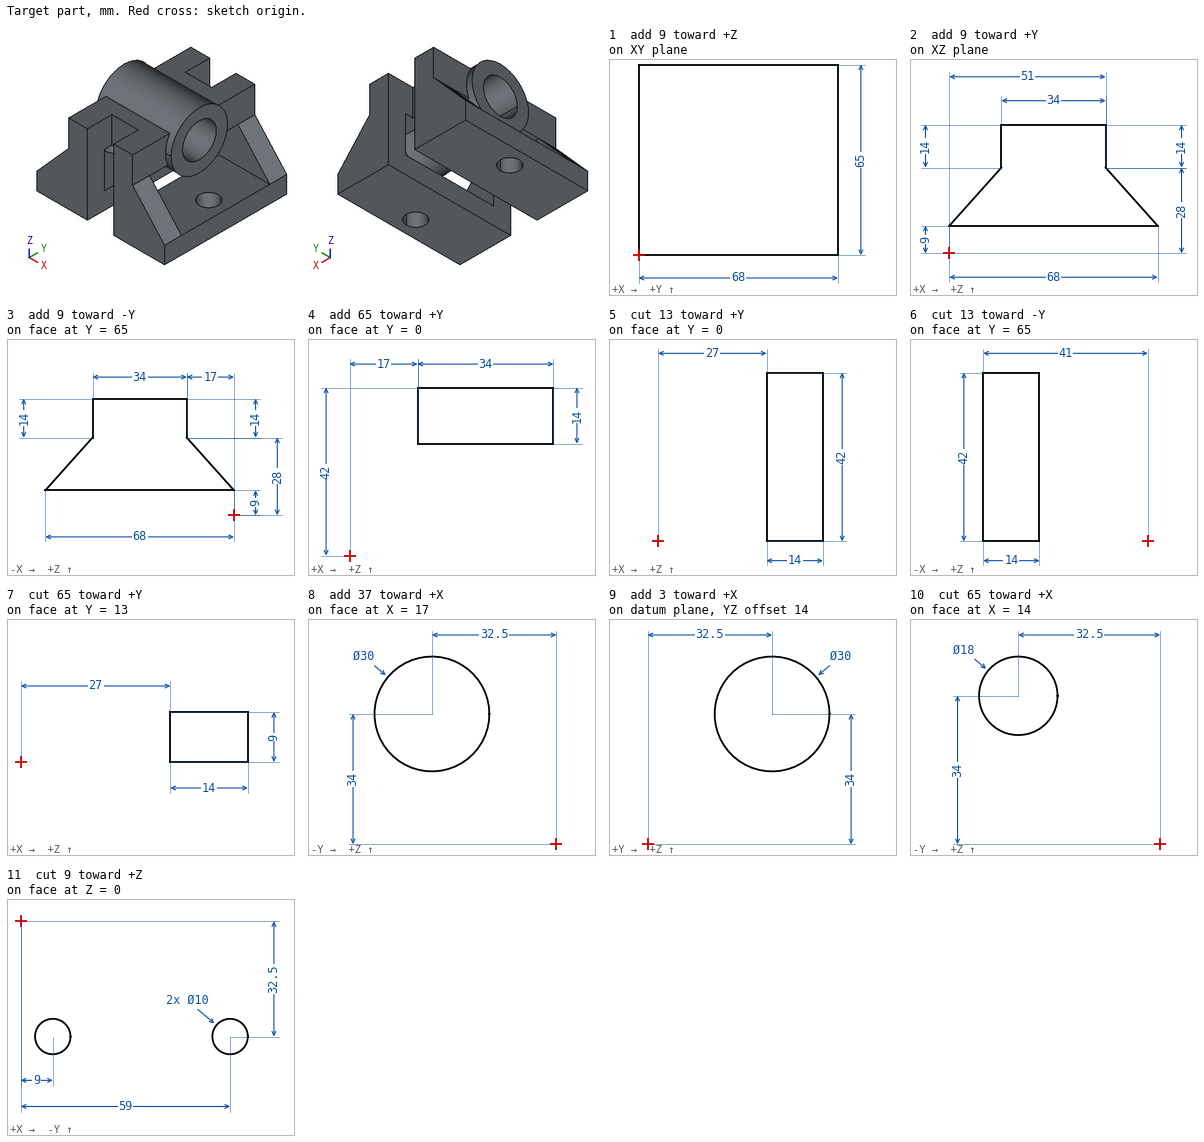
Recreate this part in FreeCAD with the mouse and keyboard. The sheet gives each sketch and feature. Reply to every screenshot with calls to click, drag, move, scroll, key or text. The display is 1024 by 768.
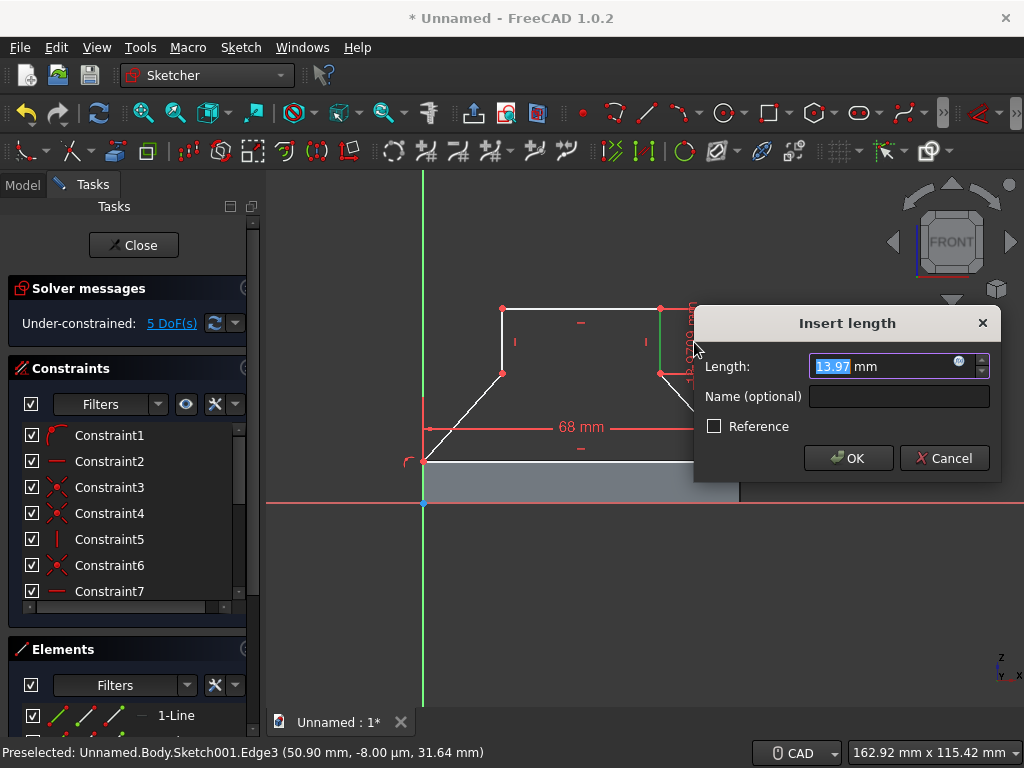
text(14)
key(Return)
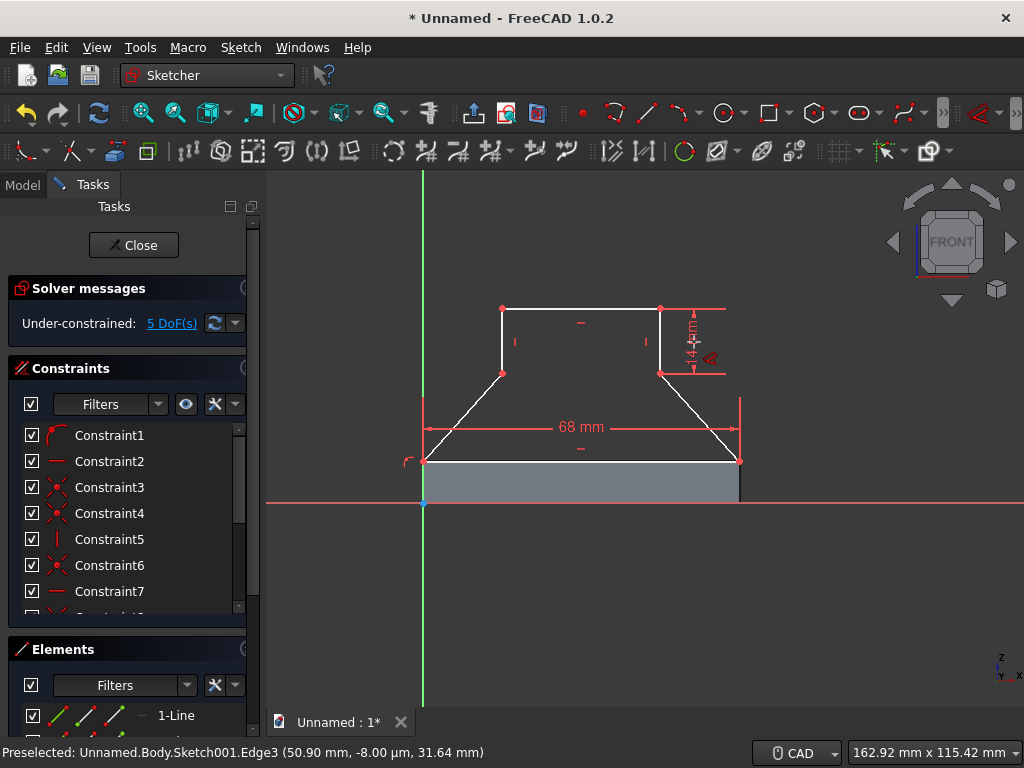
click(613, 309)
click(581, 275)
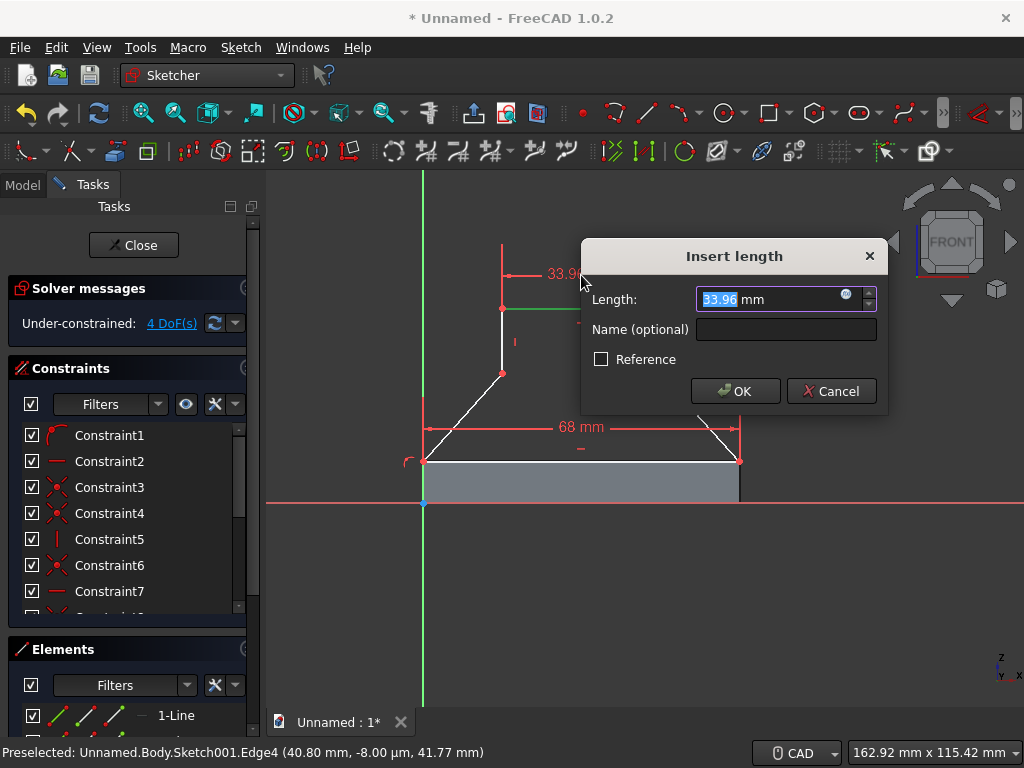
text(34)
key(Return)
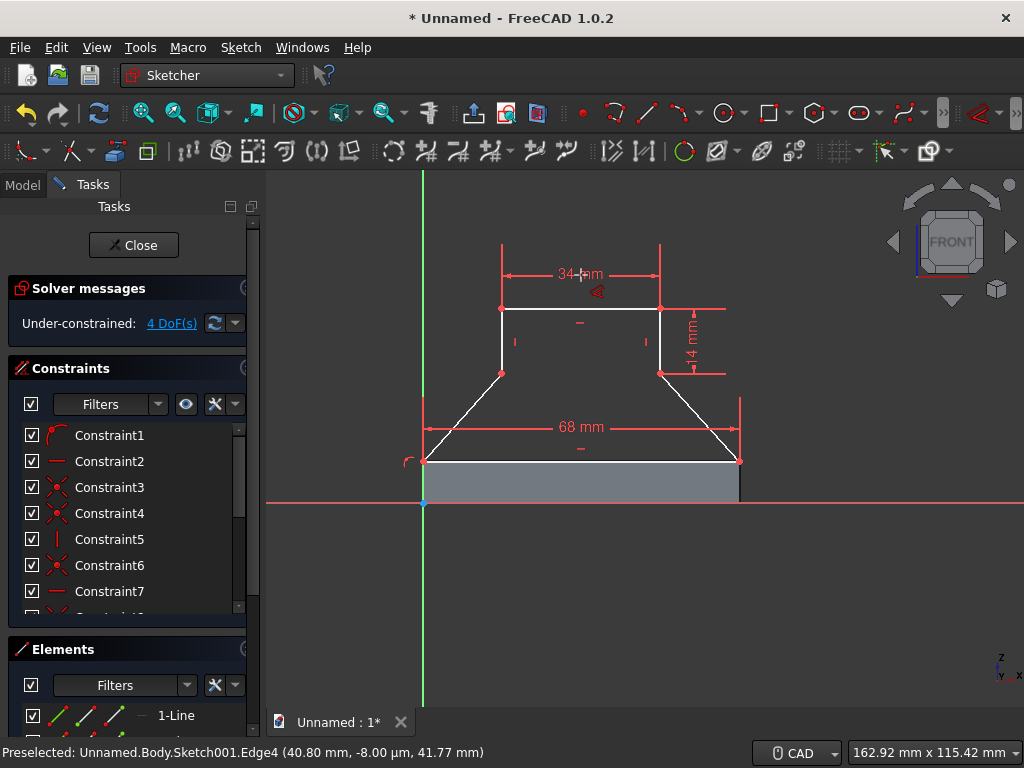
click(502, 328)
click(468, 341)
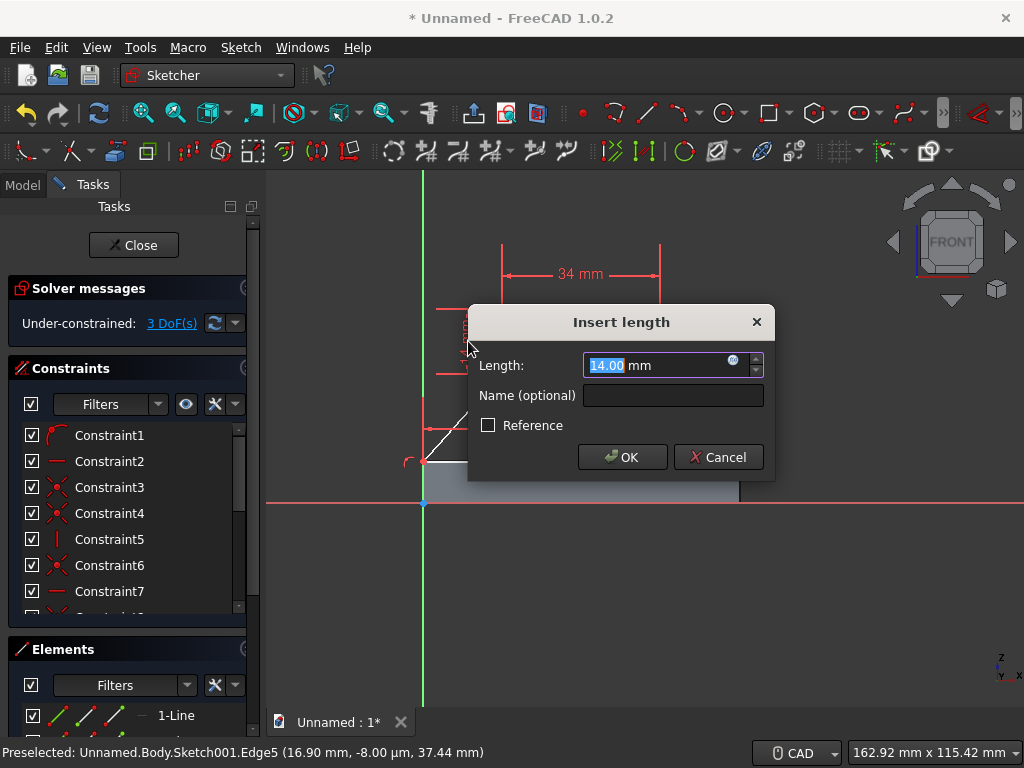
text(14)
key(Return)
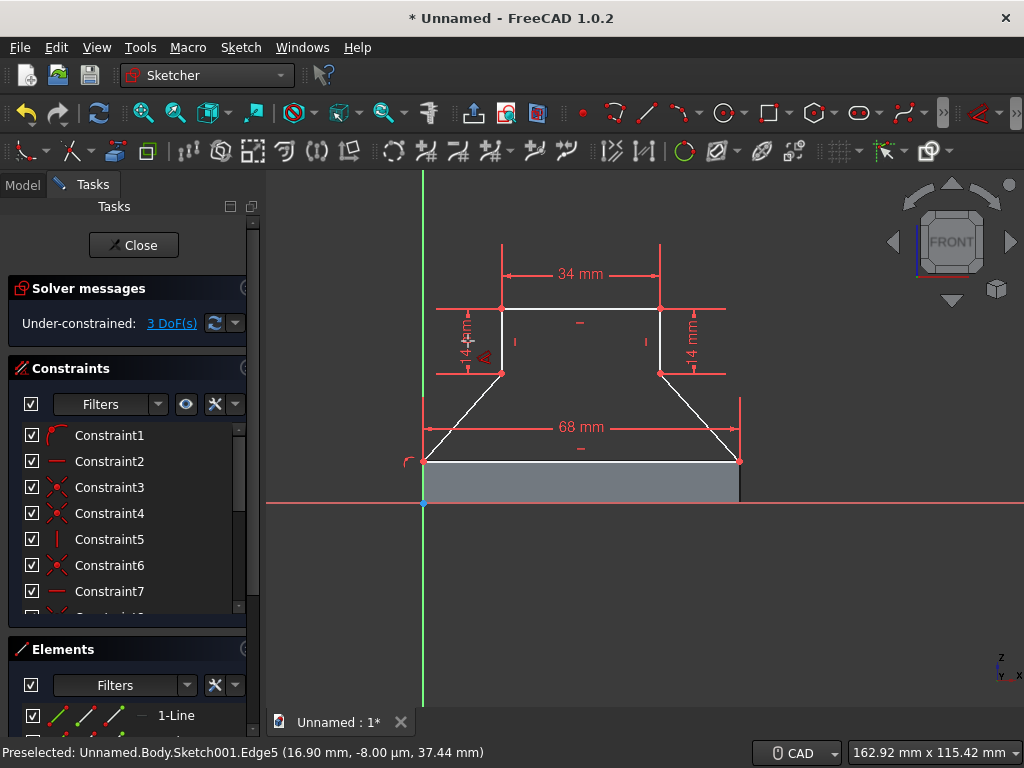
click(423, 462)
click(389, 483)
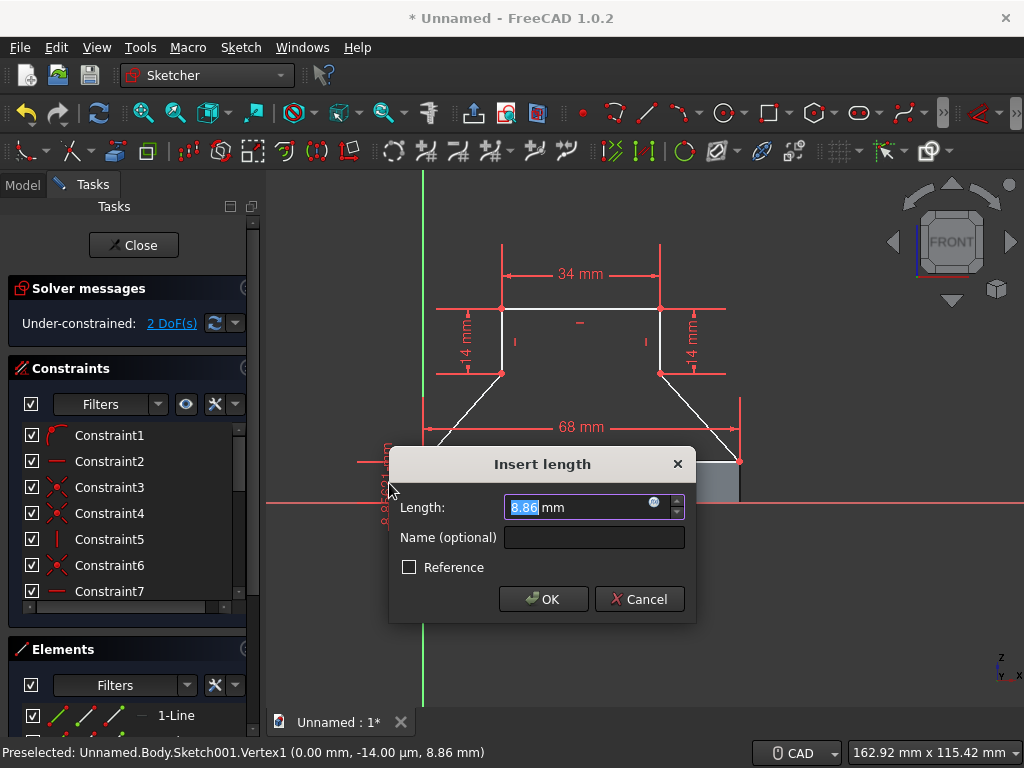
text(9)
key(Return)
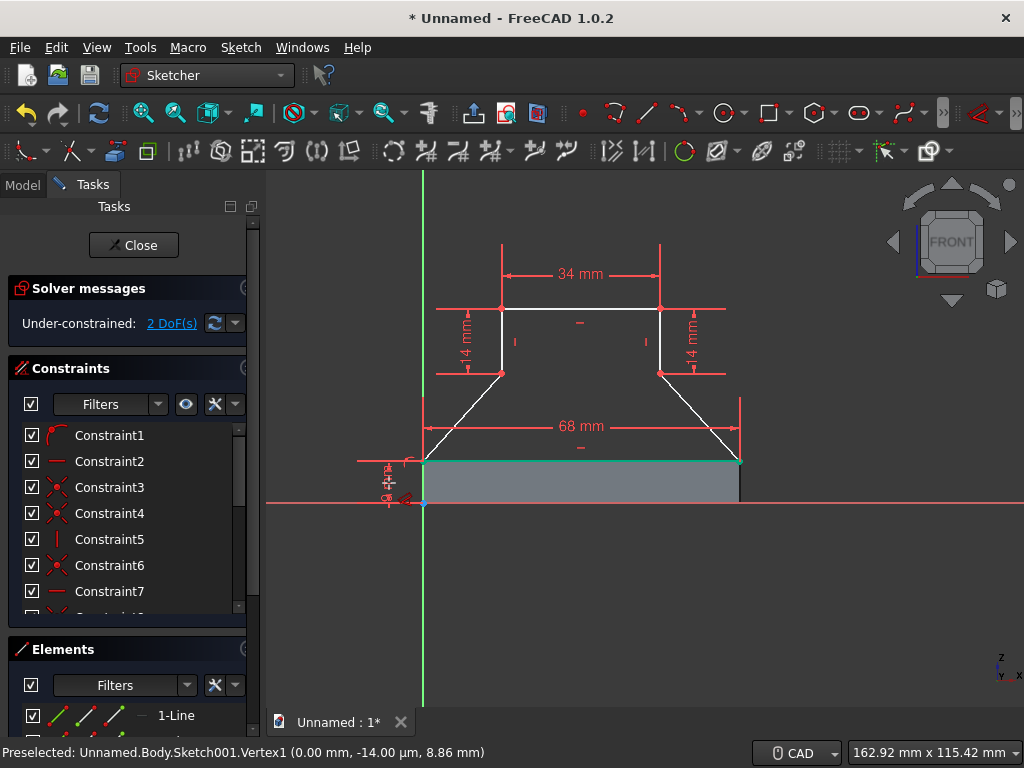
click(660, 374)
click(542, 537)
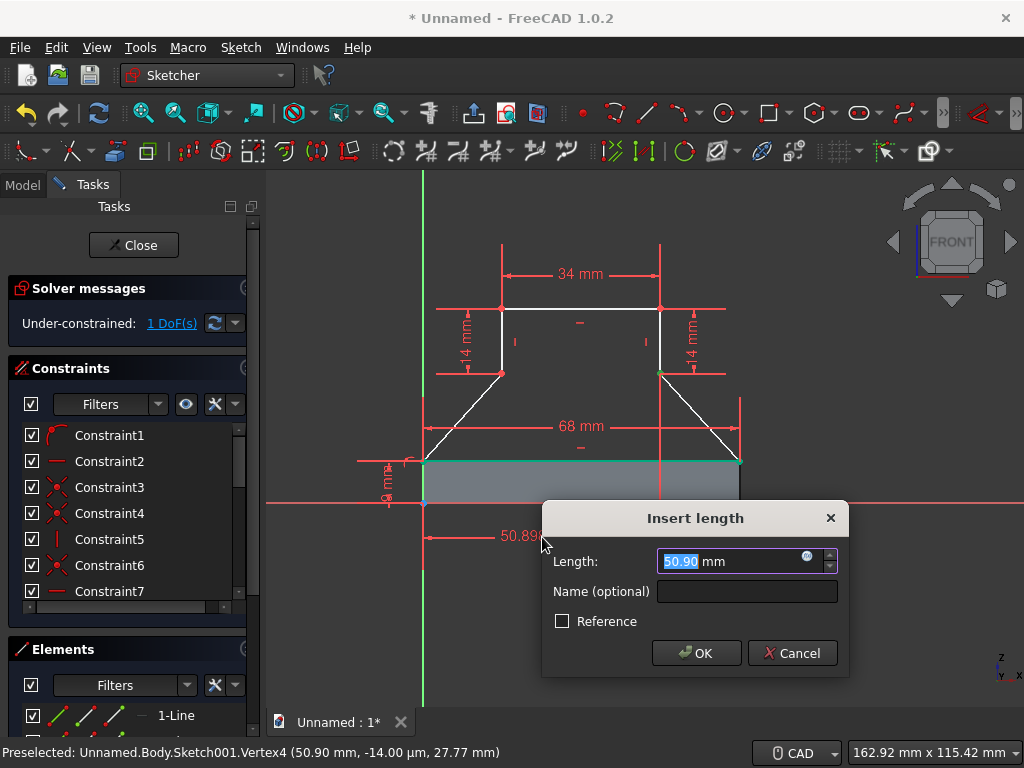
text(51)
key(Return)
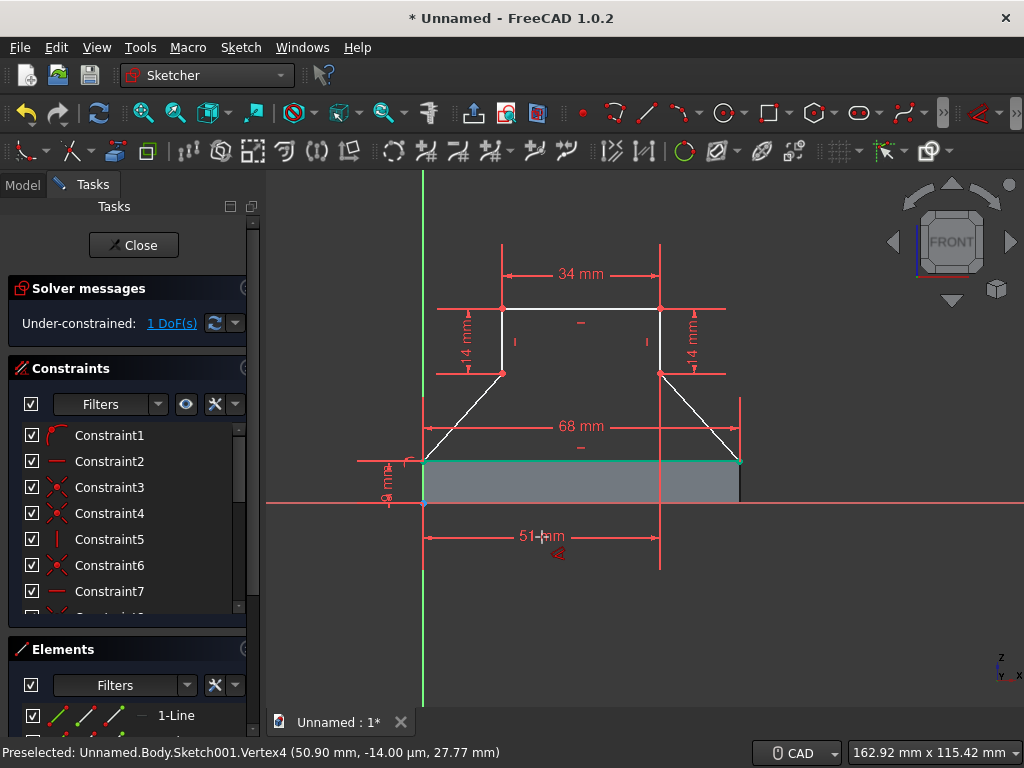
click(660, 374)
click(389, 439)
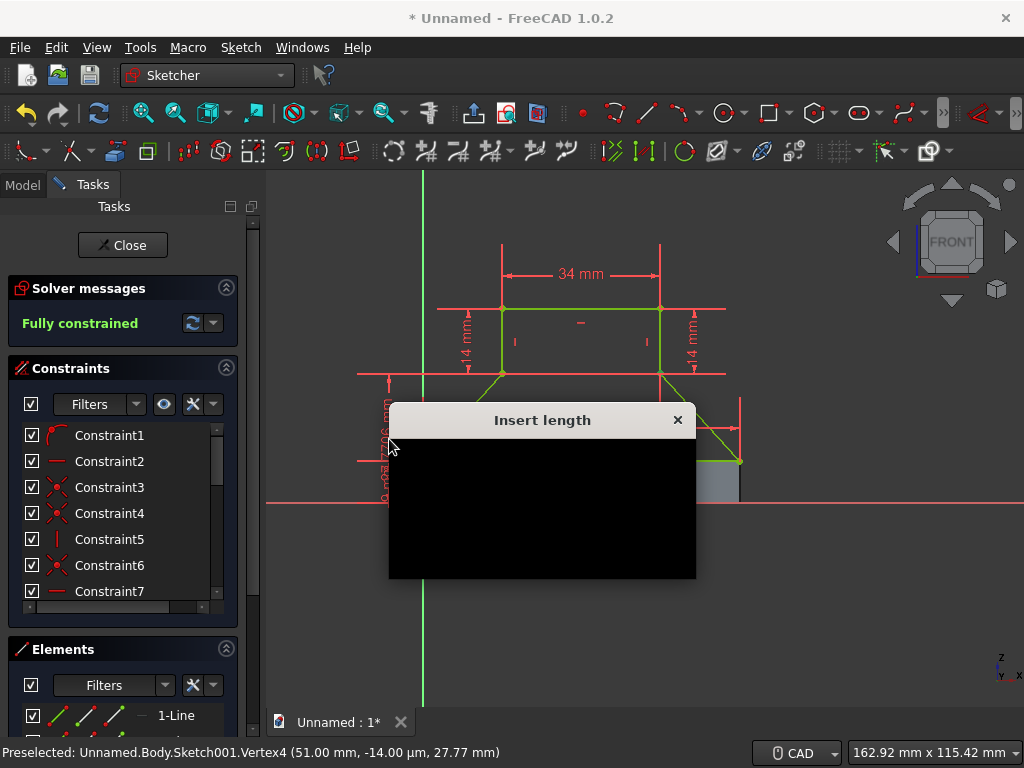
text(28)
key(Return)
key(Escape)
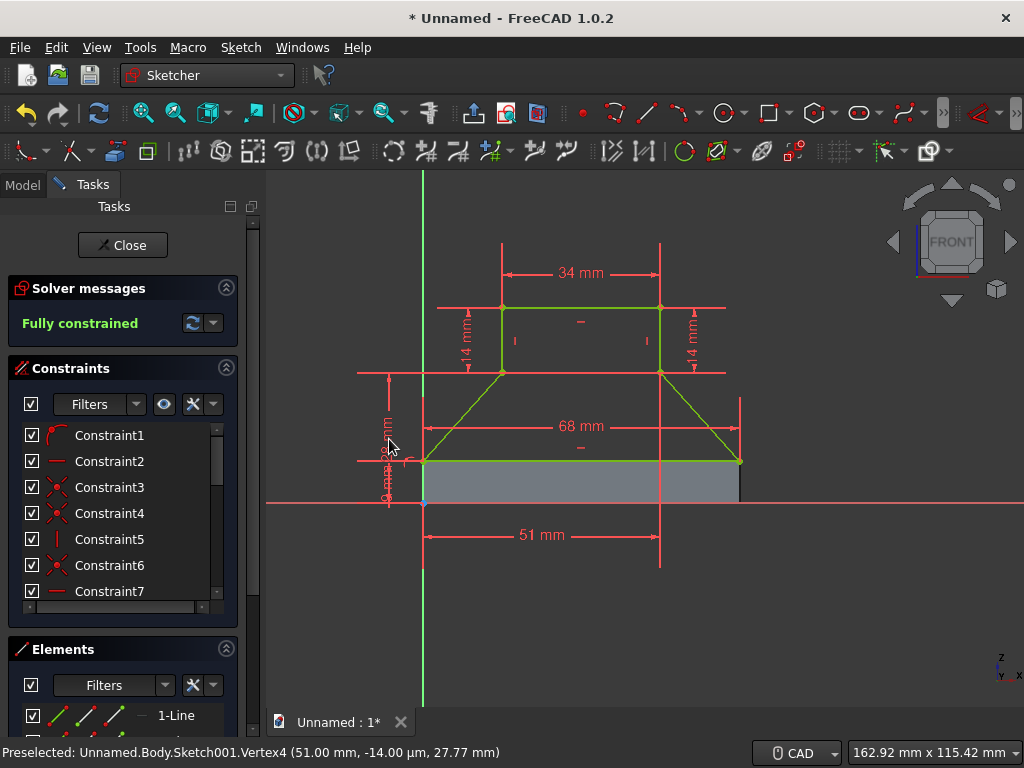
click(123, 245)